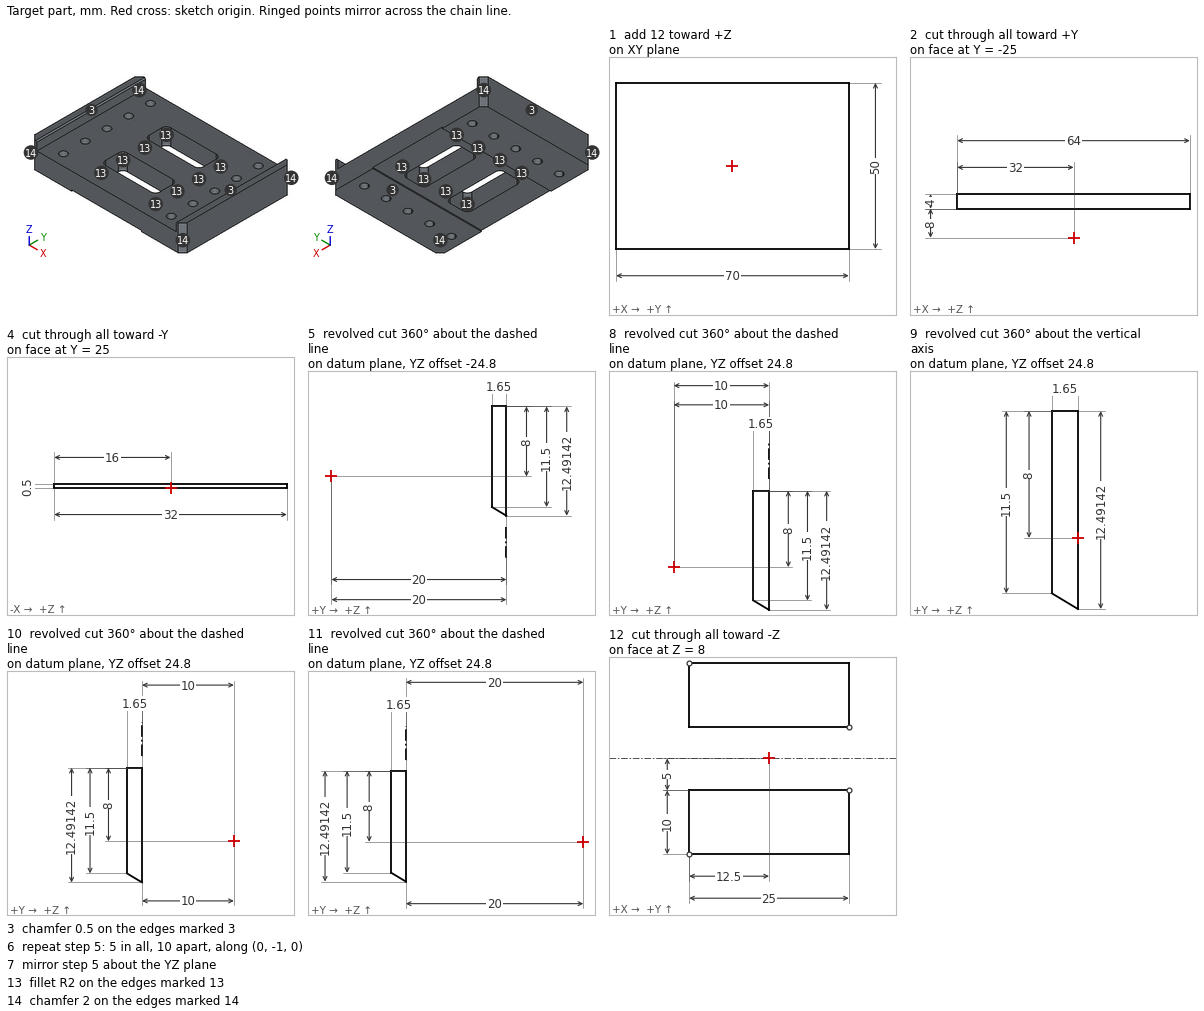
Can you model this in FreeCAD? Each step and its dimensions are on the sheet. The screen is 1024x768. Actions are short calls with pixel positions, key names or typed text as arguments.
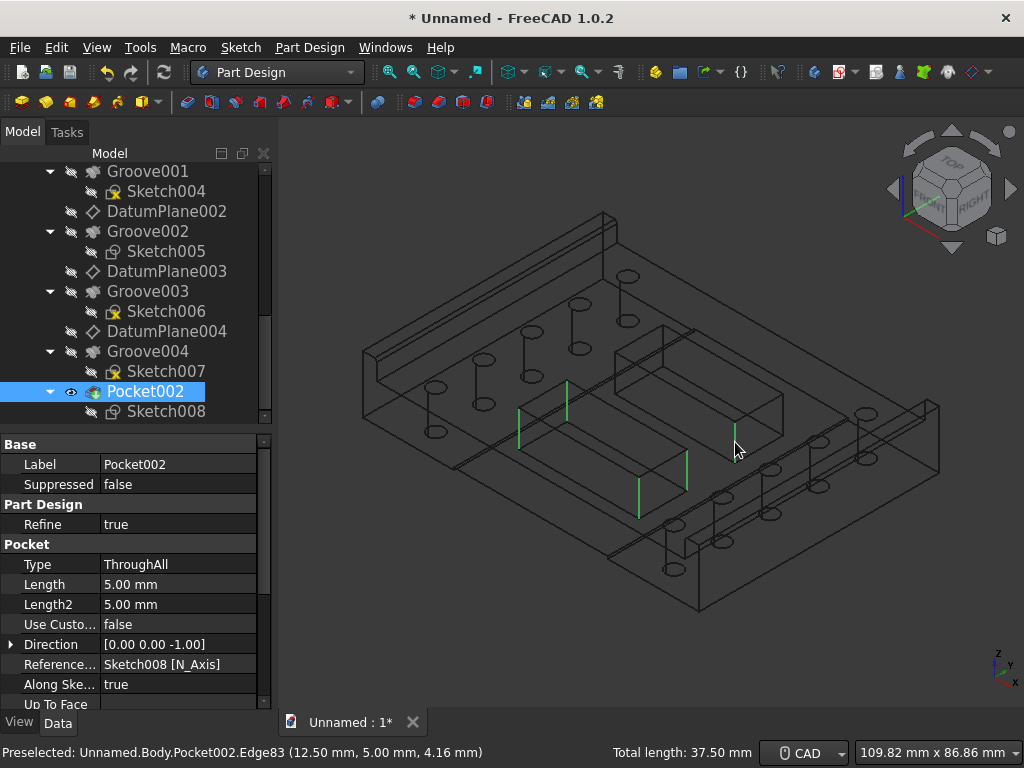
click(615, 372, ctrl)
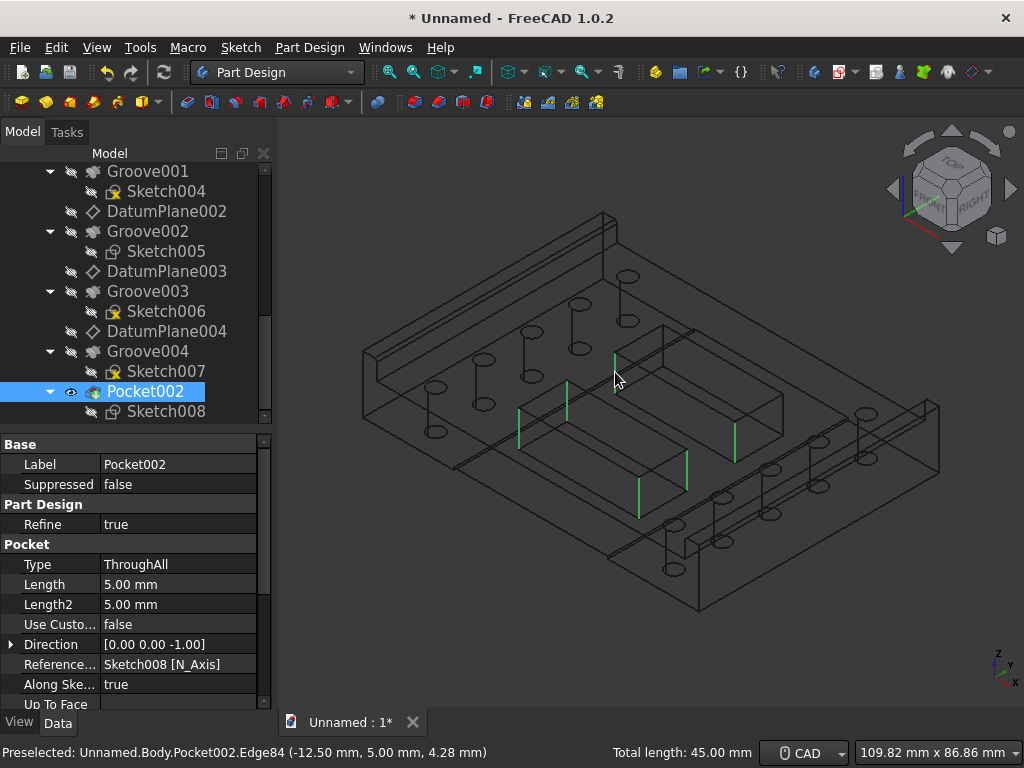
click(663, 344, ctrl)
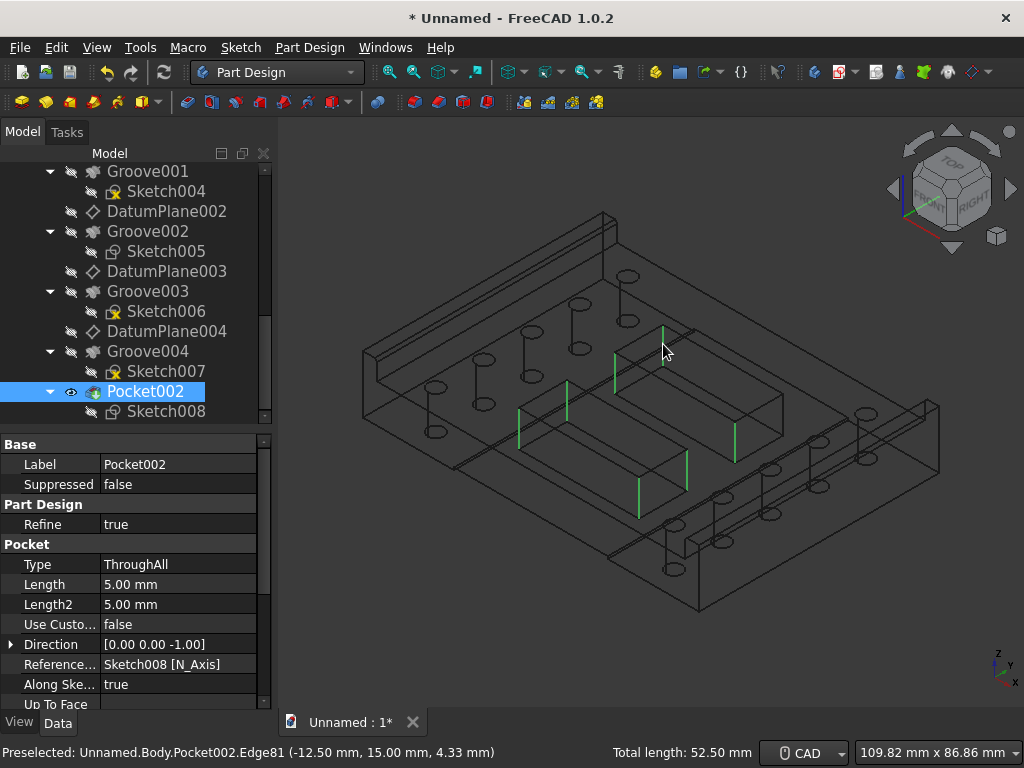
click(783, 414, ctrl)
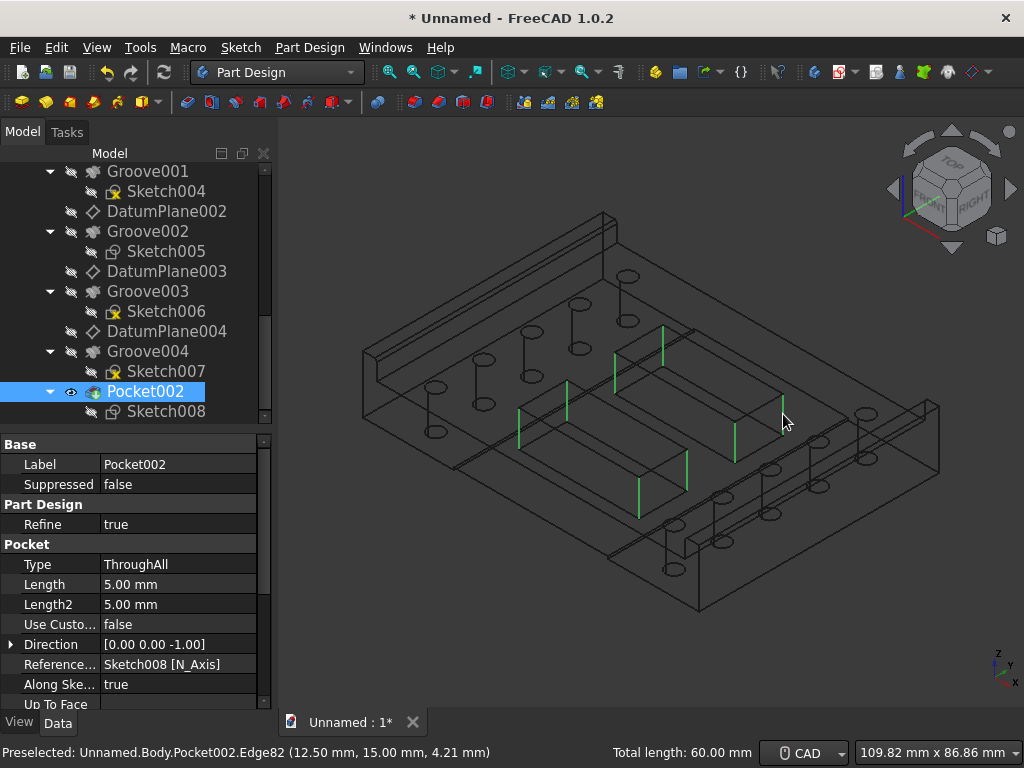
key(v)
key(1)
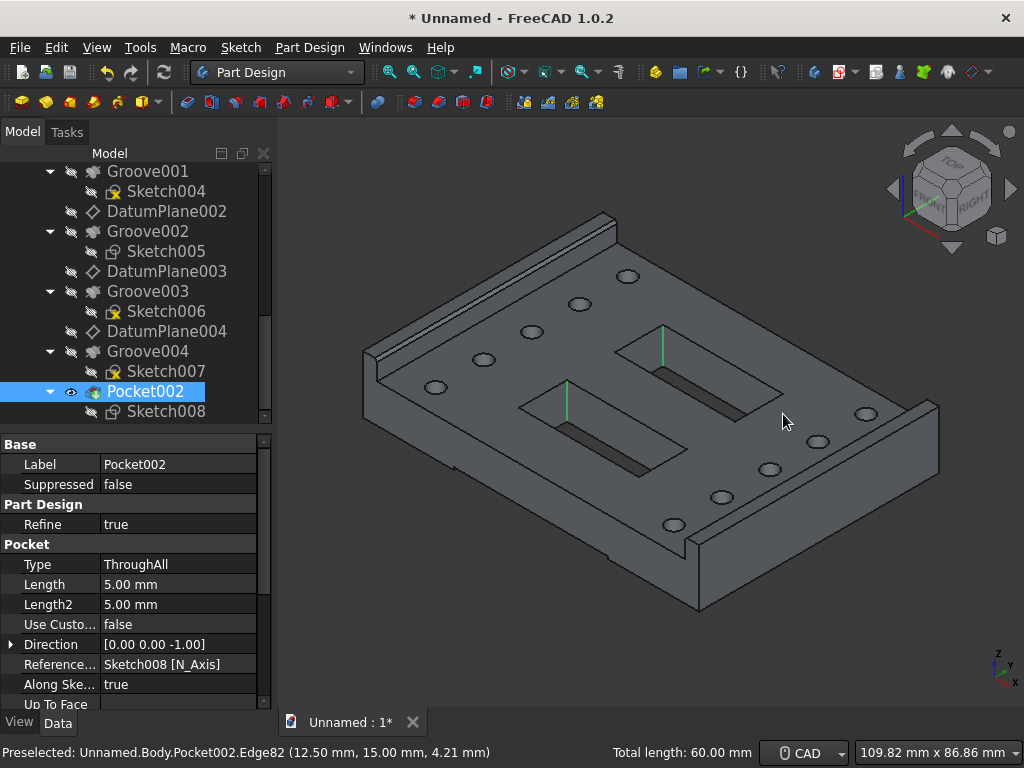
click(416, 102)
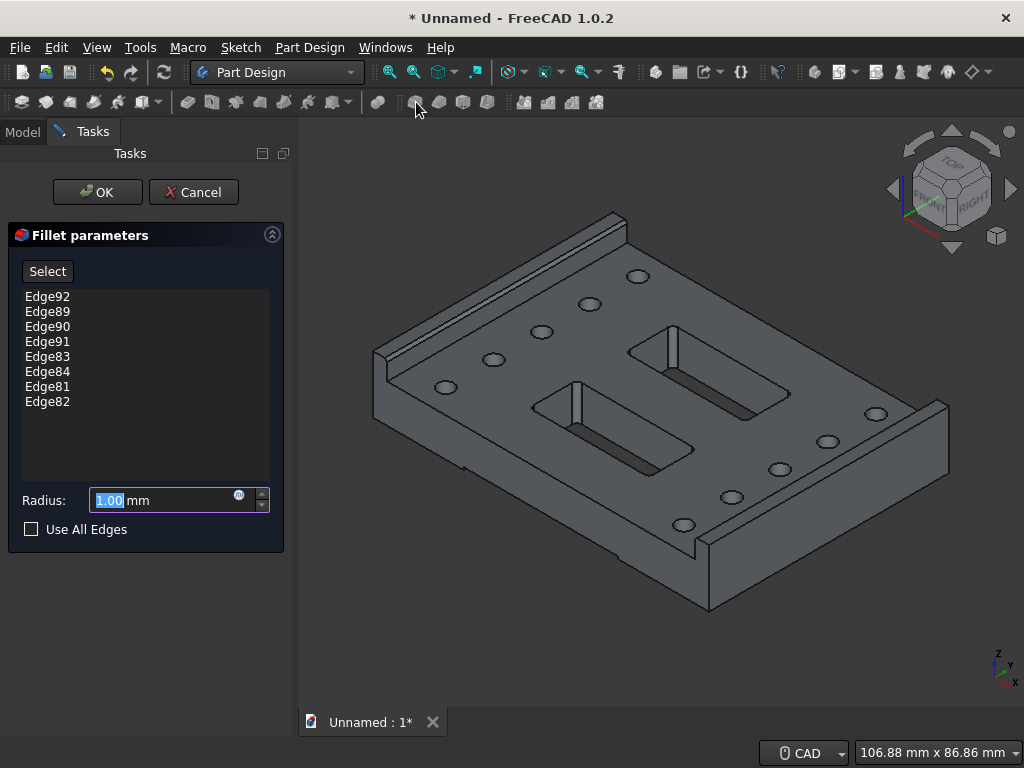
text(2)
key(Tab)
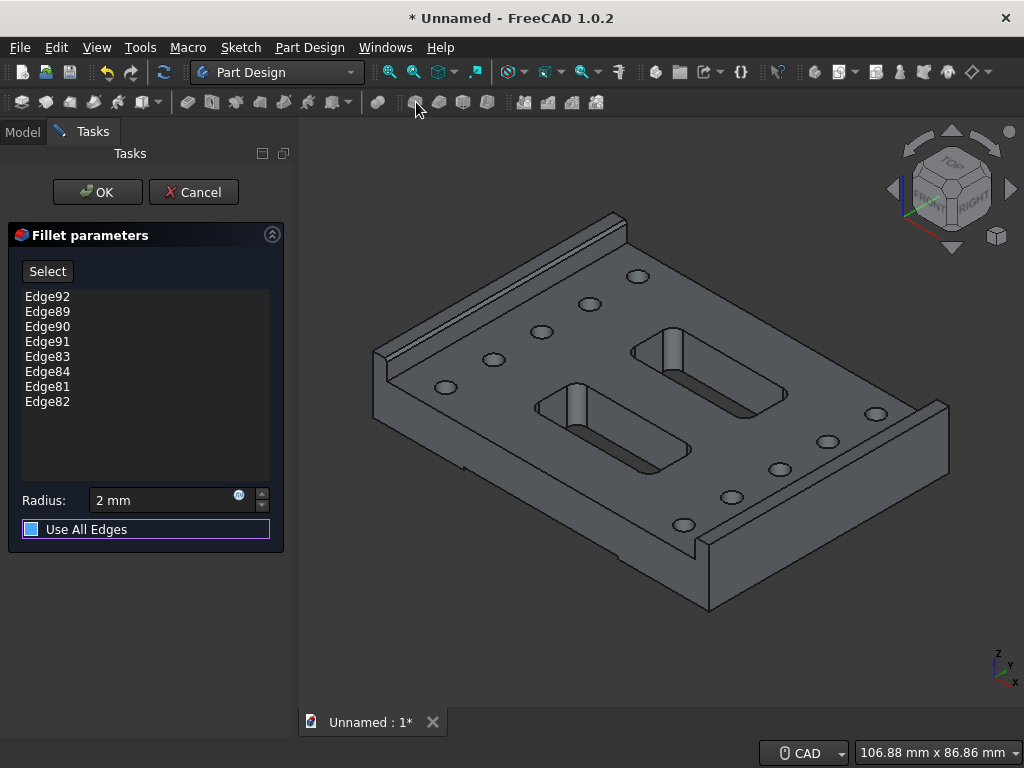
click(98, 192)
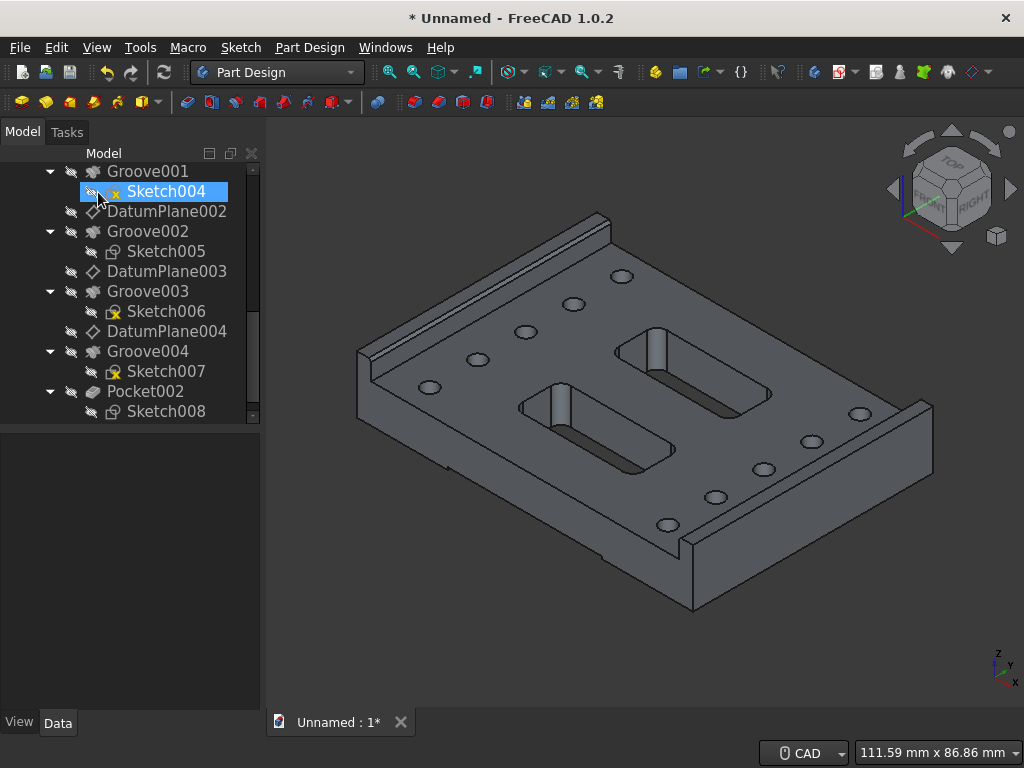
click(693, 577)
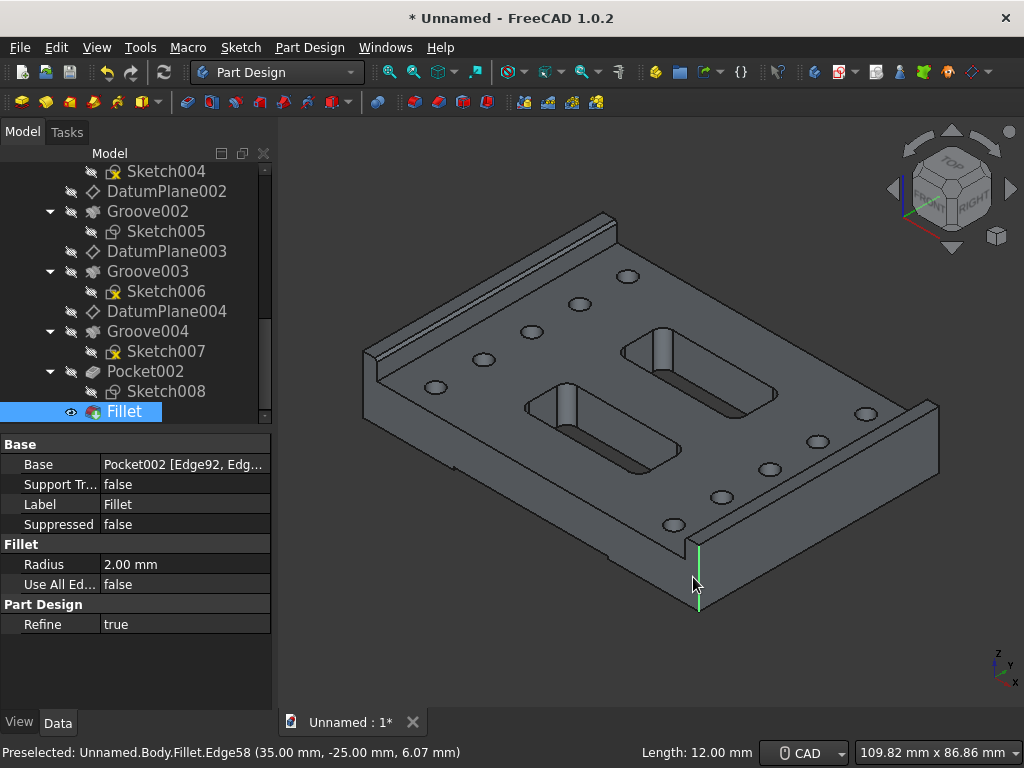
key(2)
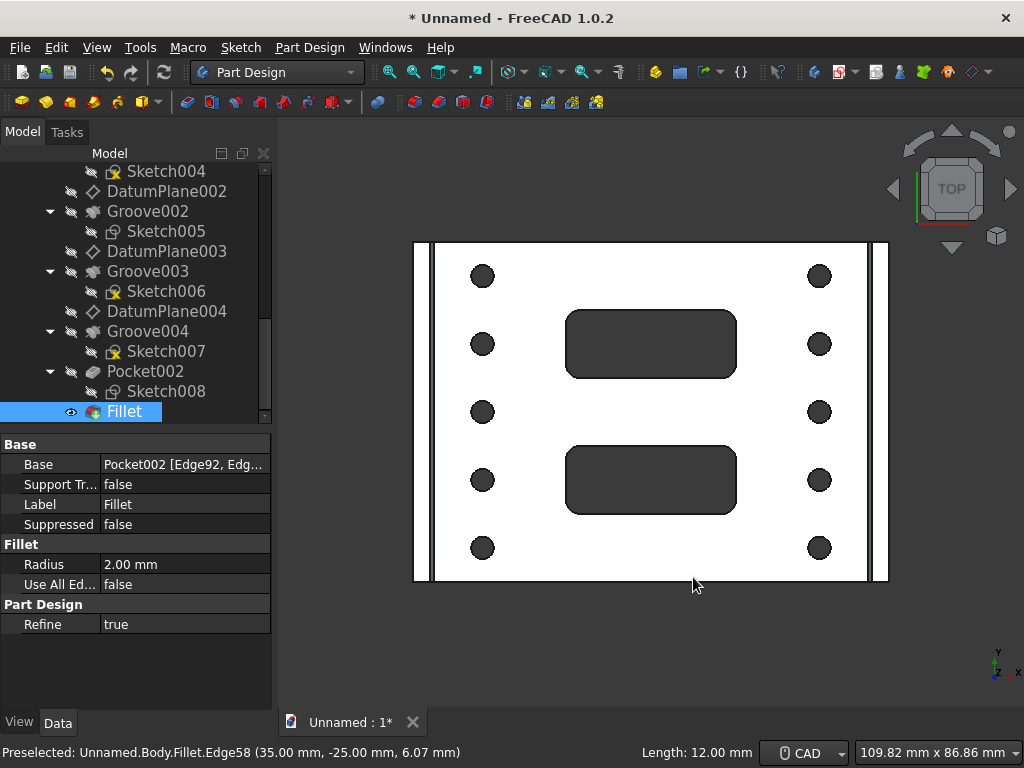
key(0)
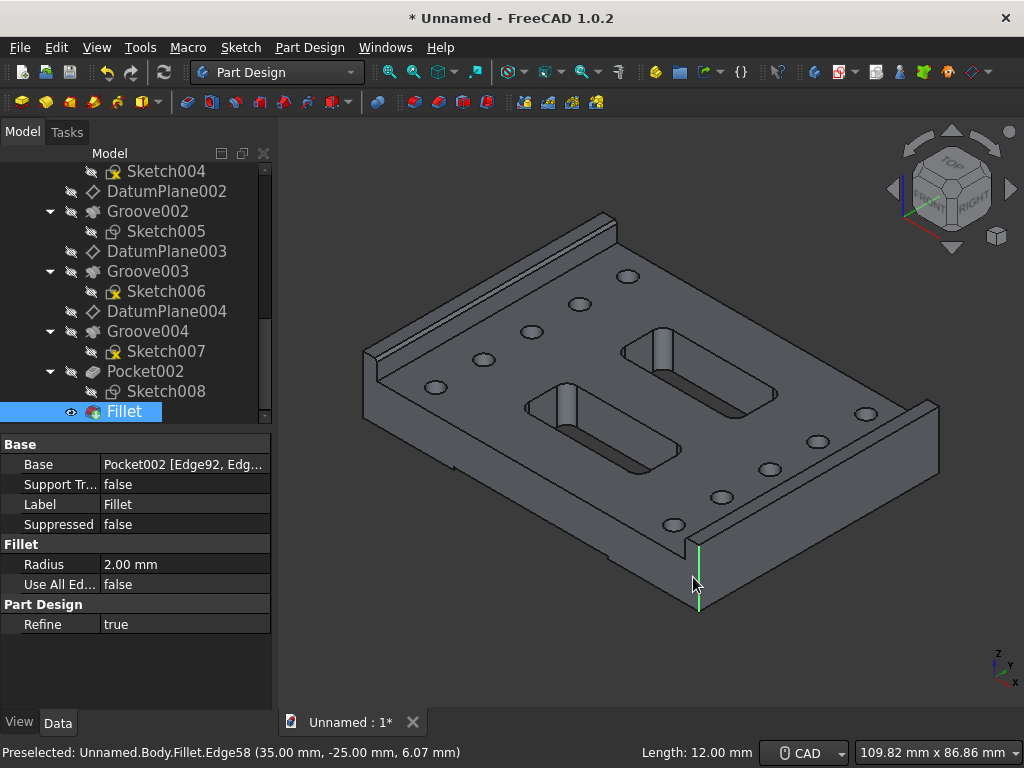
key(1)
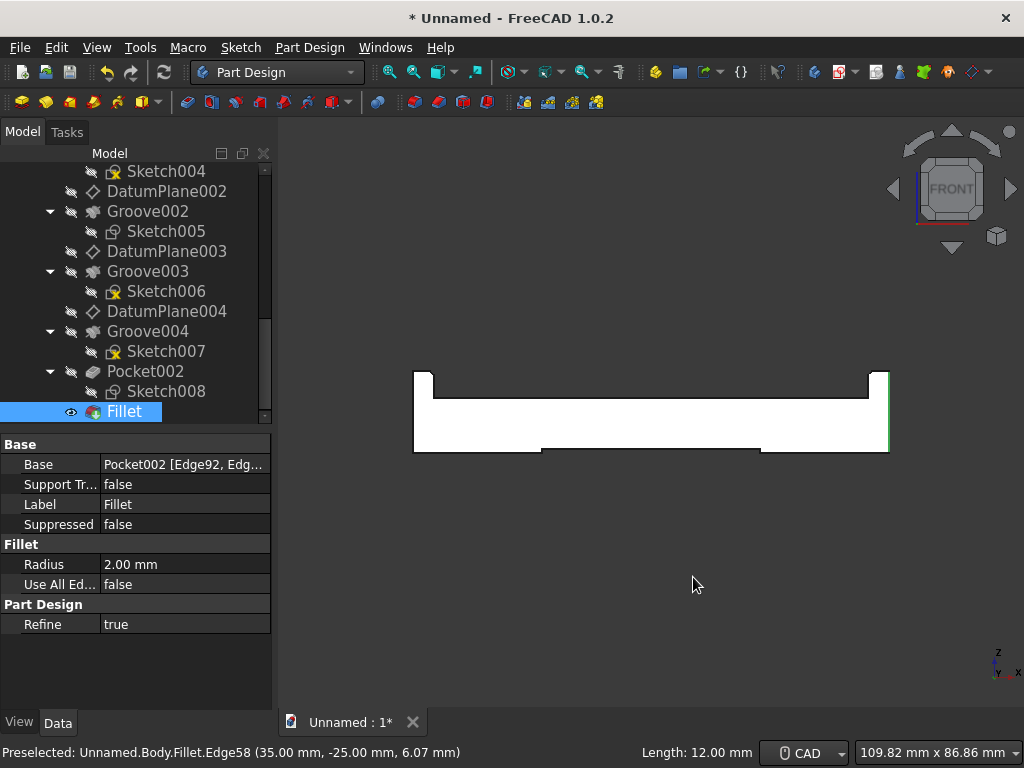
click(413, 411, ctrl)